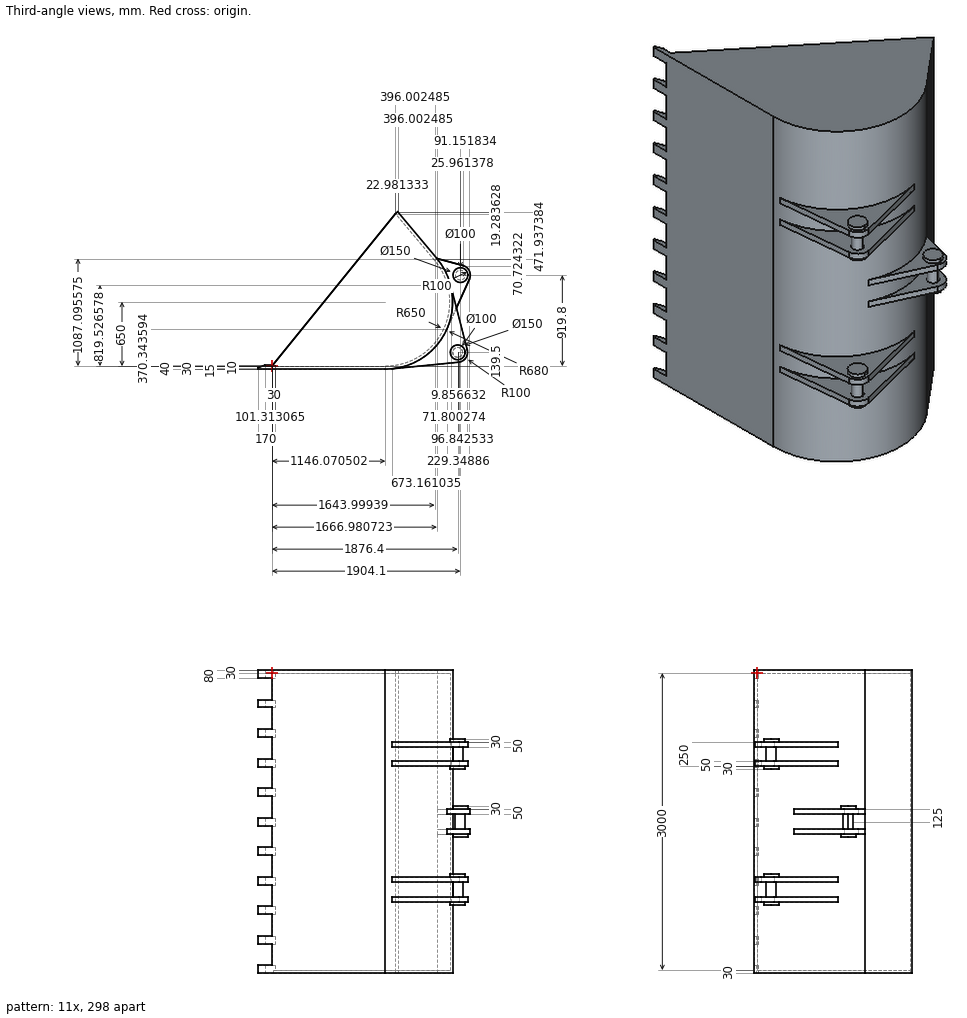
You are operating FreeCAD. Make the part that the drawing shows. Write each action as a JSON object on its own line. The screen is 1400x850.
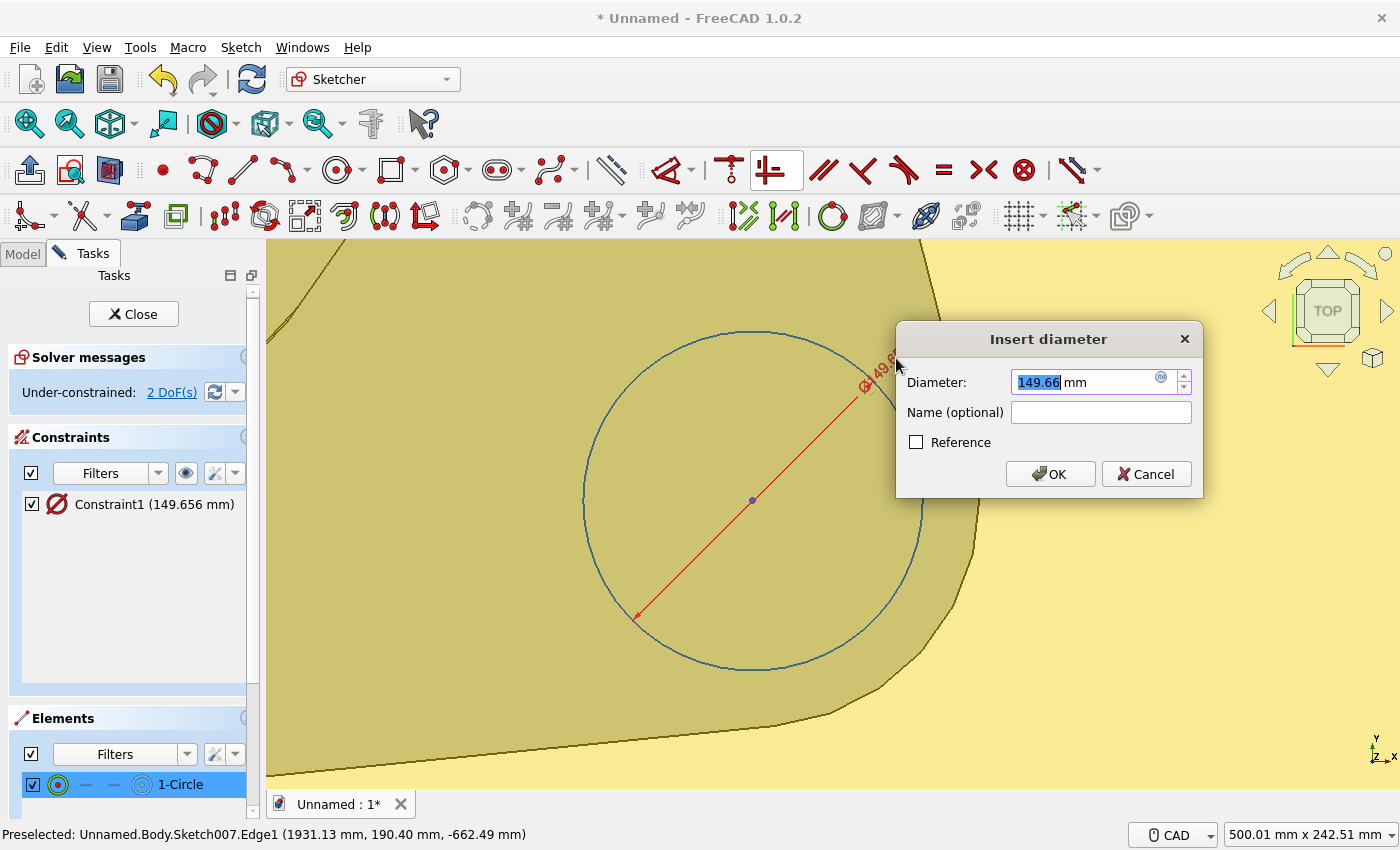
{"action": "type", "text": "150"}
{"action": "key", "text": "Return"}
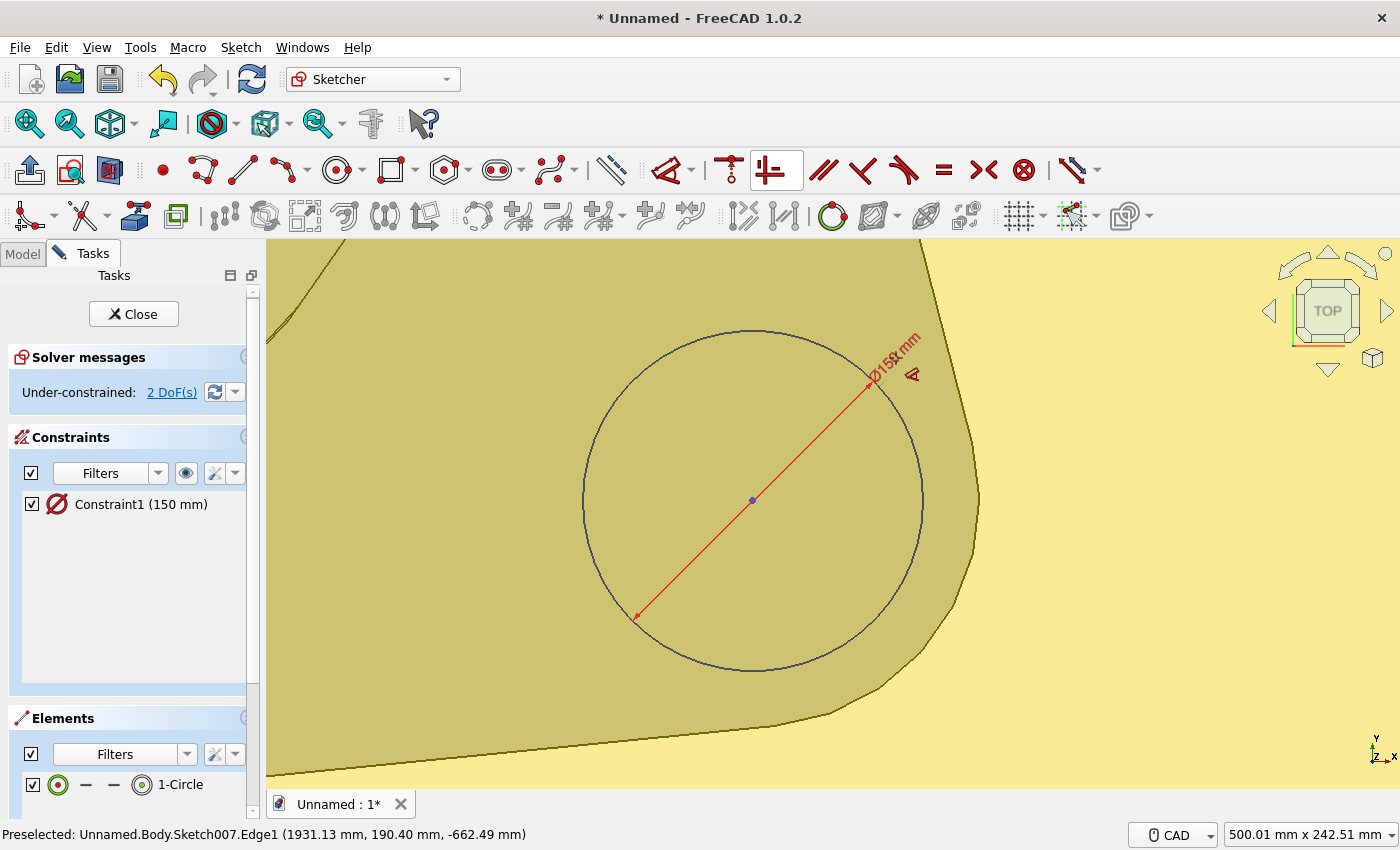
{"action": "left_click", "coordinate": [753, 501]}
{"action": "left_click", "coordinate": [787, 631]}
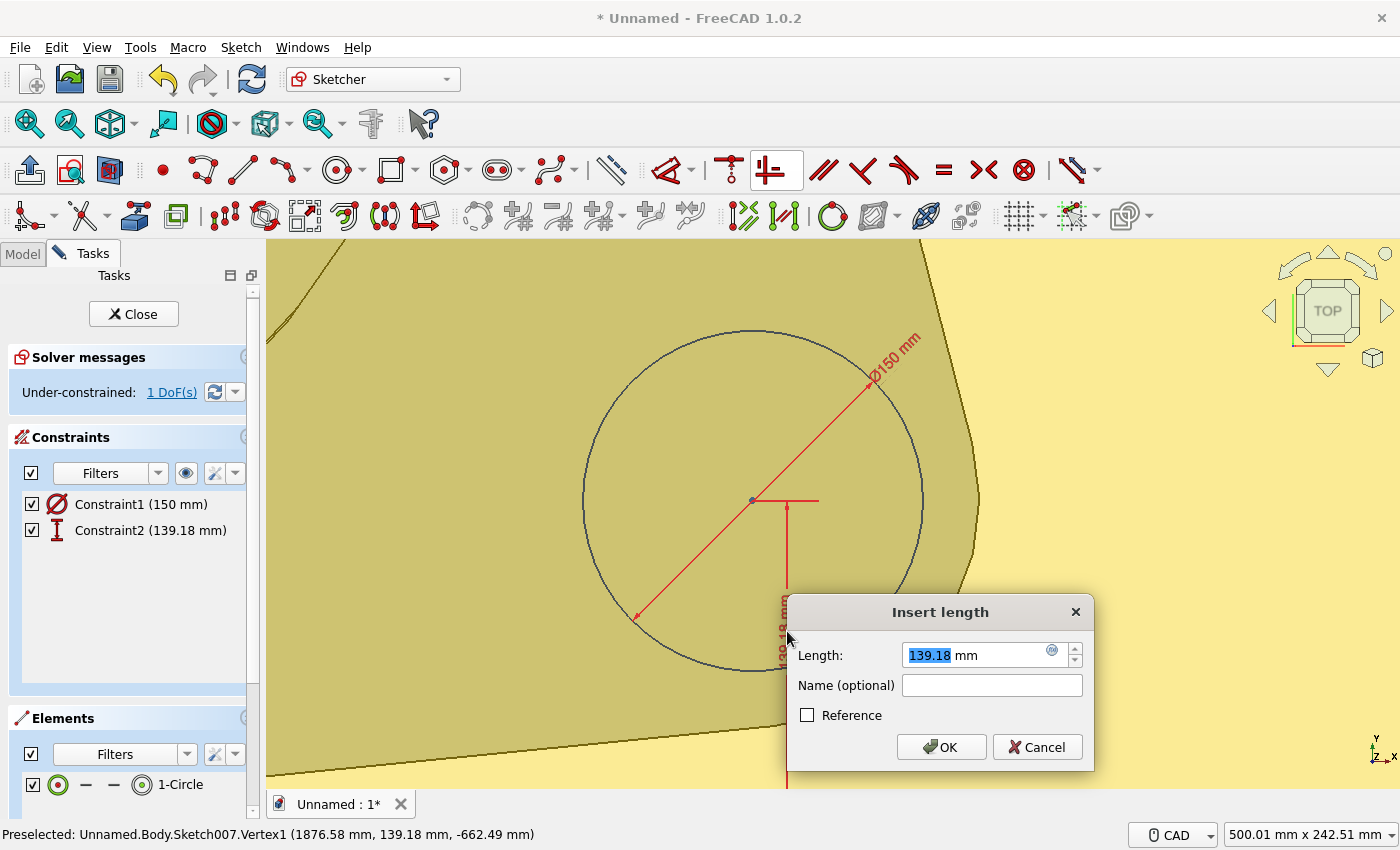
{"action": "type", "text": "139.5"}
{"action": "key", "text": "Return"}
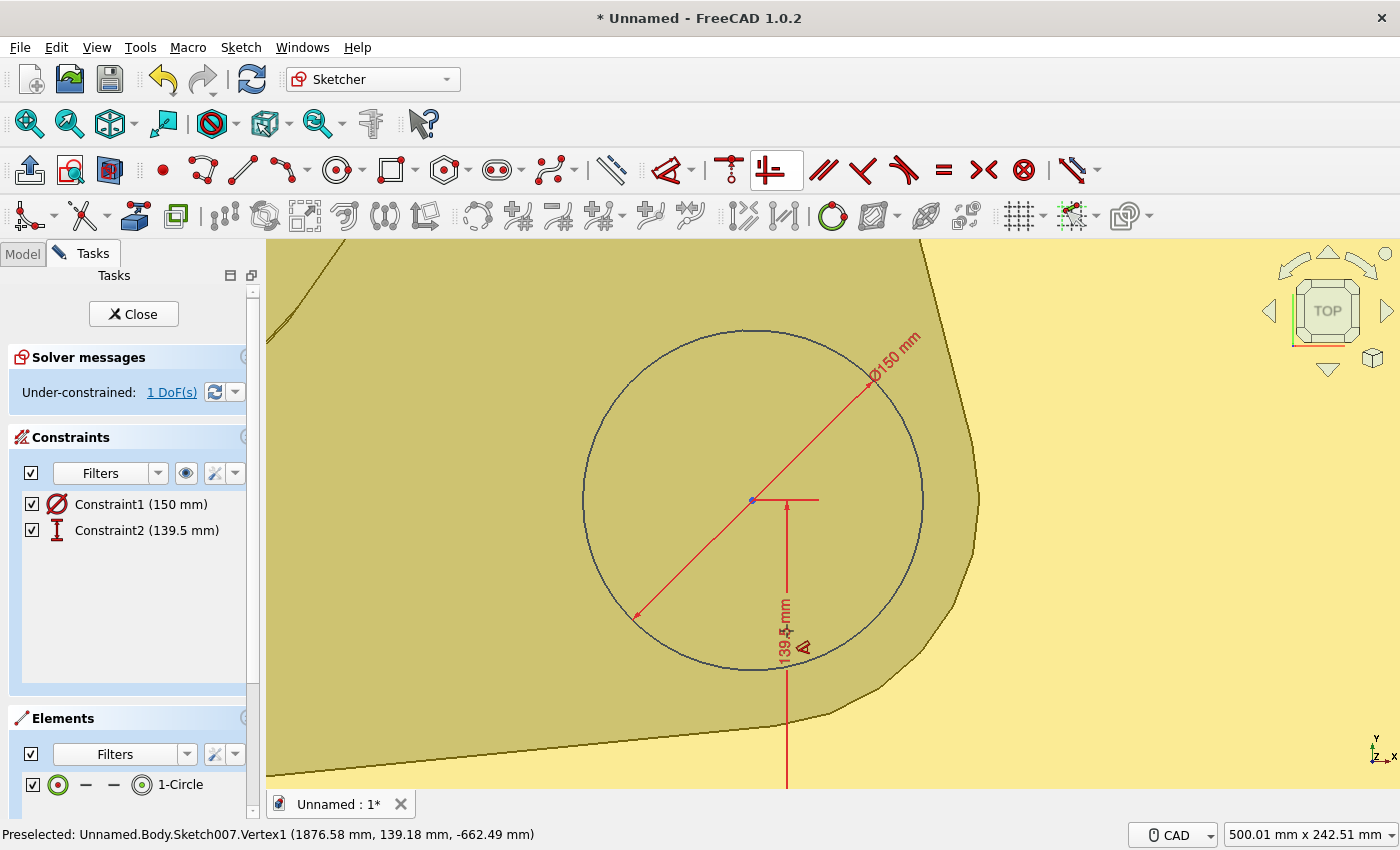
{"action": "left_click", "coordinate": [753, 500]}
{"action": "left_click", "coordinate": [523, 466]}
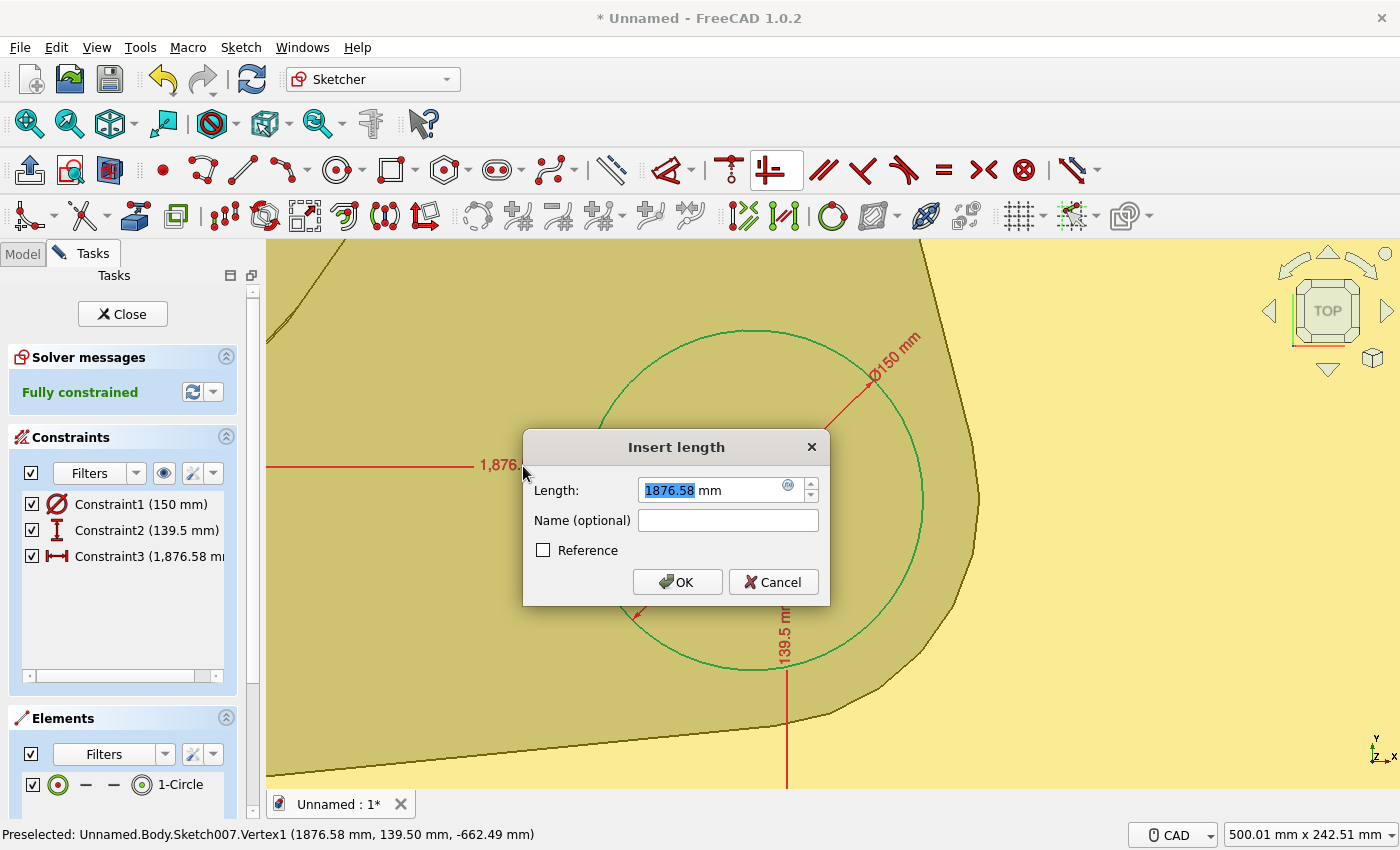
{"action": "type", "text": "1876.4"}
{"action": "key", "text": "Return"}
{"action": "key", "text": "Escape"}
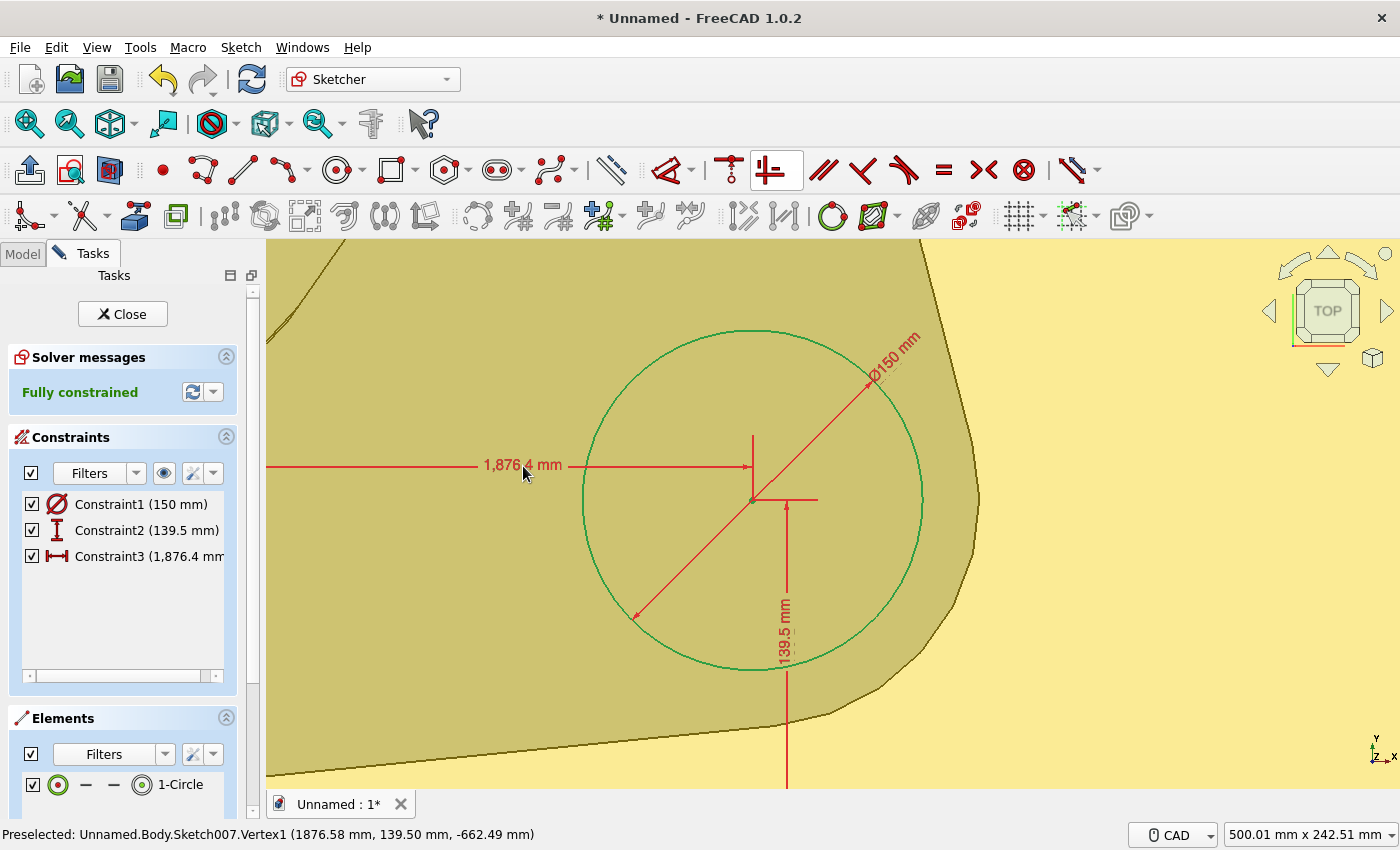
{"action": "left_click", "coordinate": [123, 314]}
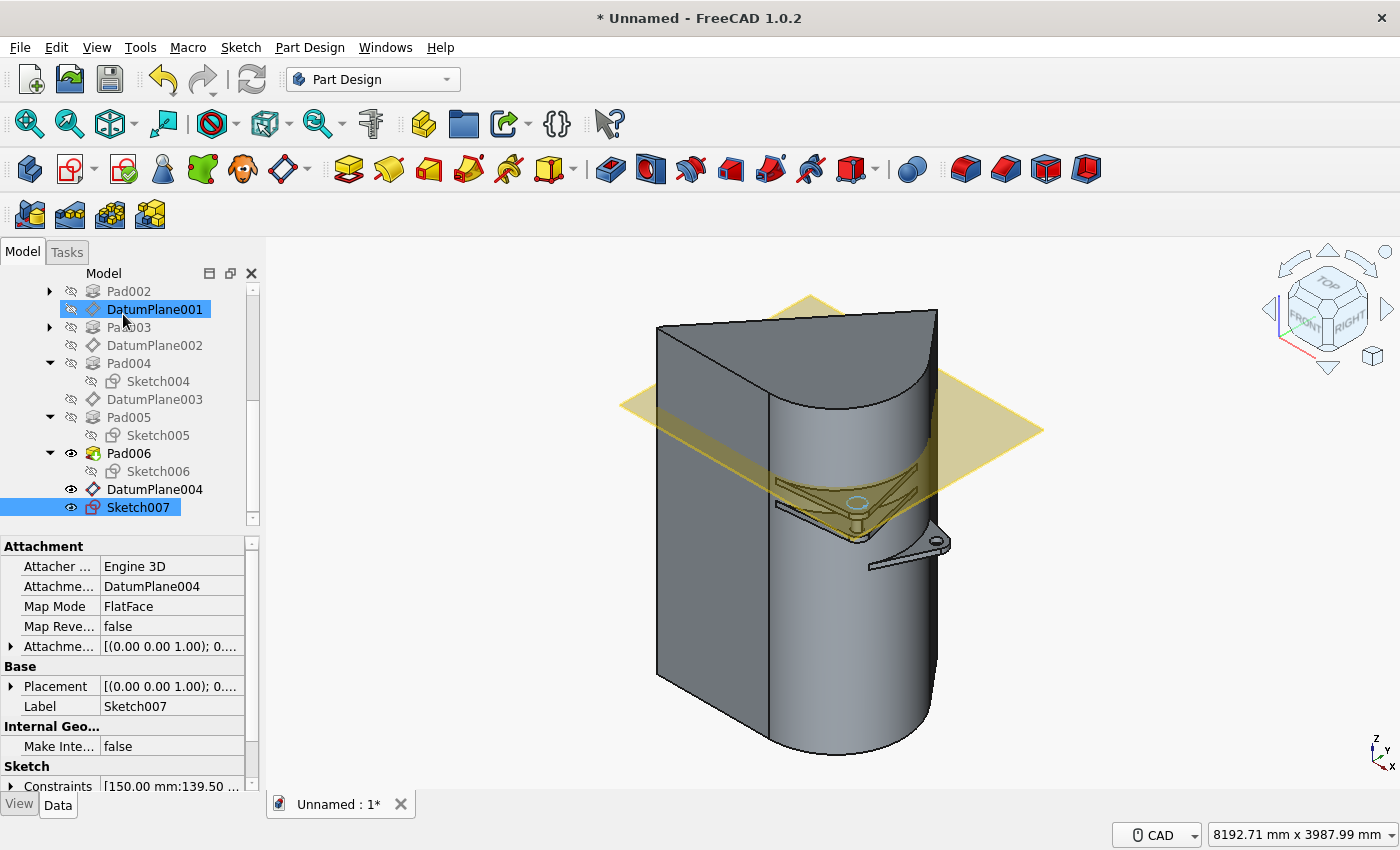
{"action": "left_click", "coordinate": [350, 170]}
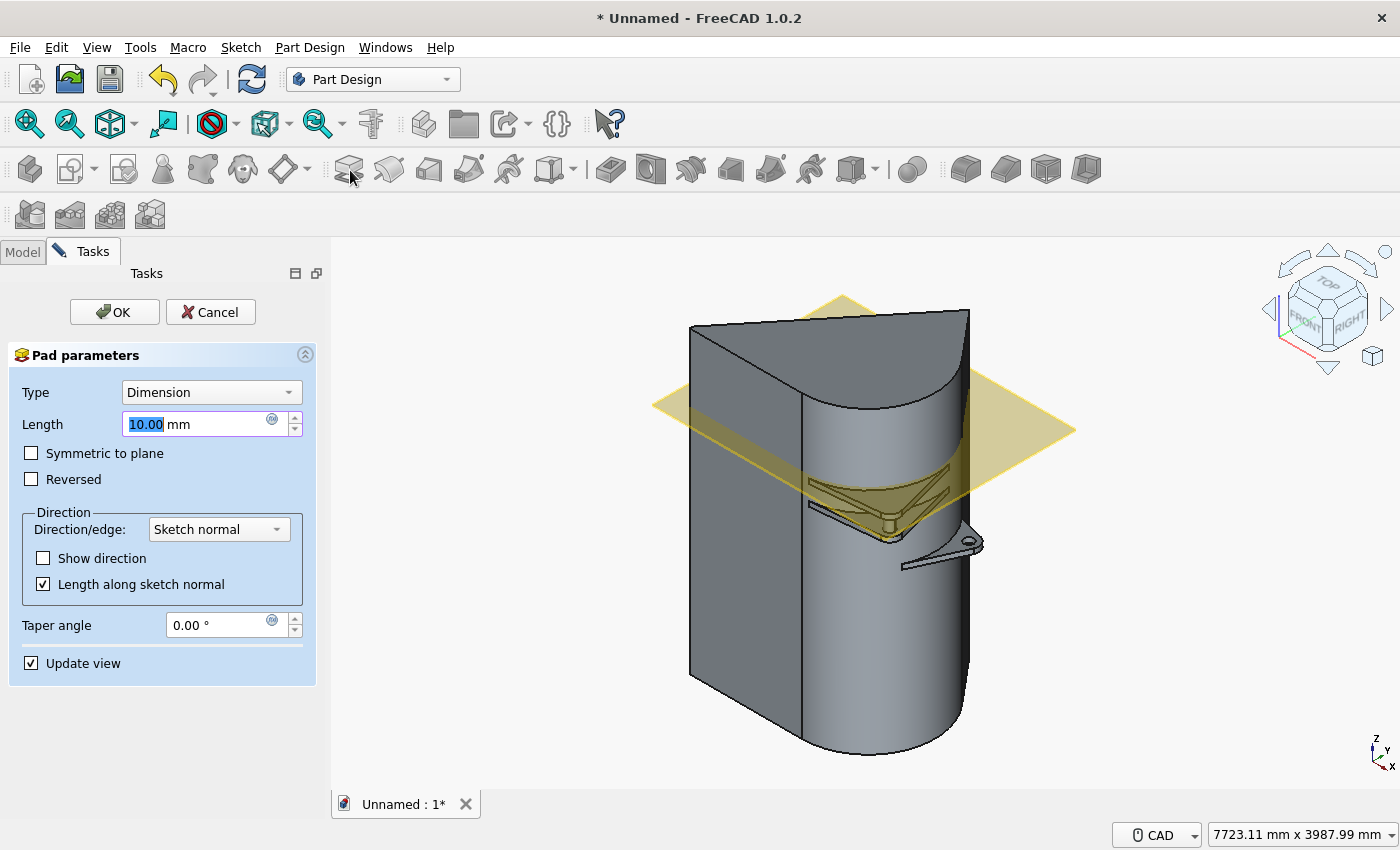
{"action": "type", "text": "30"}
{"action": "key", "text": "Tab"}